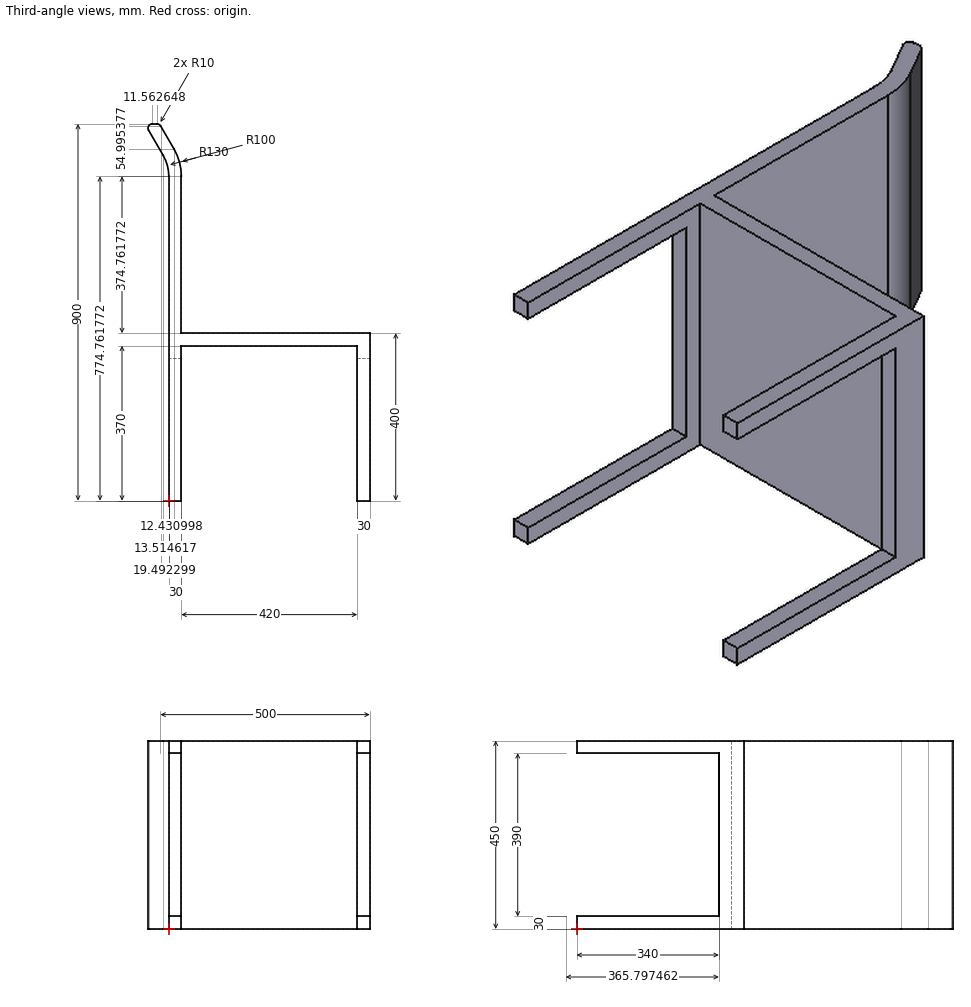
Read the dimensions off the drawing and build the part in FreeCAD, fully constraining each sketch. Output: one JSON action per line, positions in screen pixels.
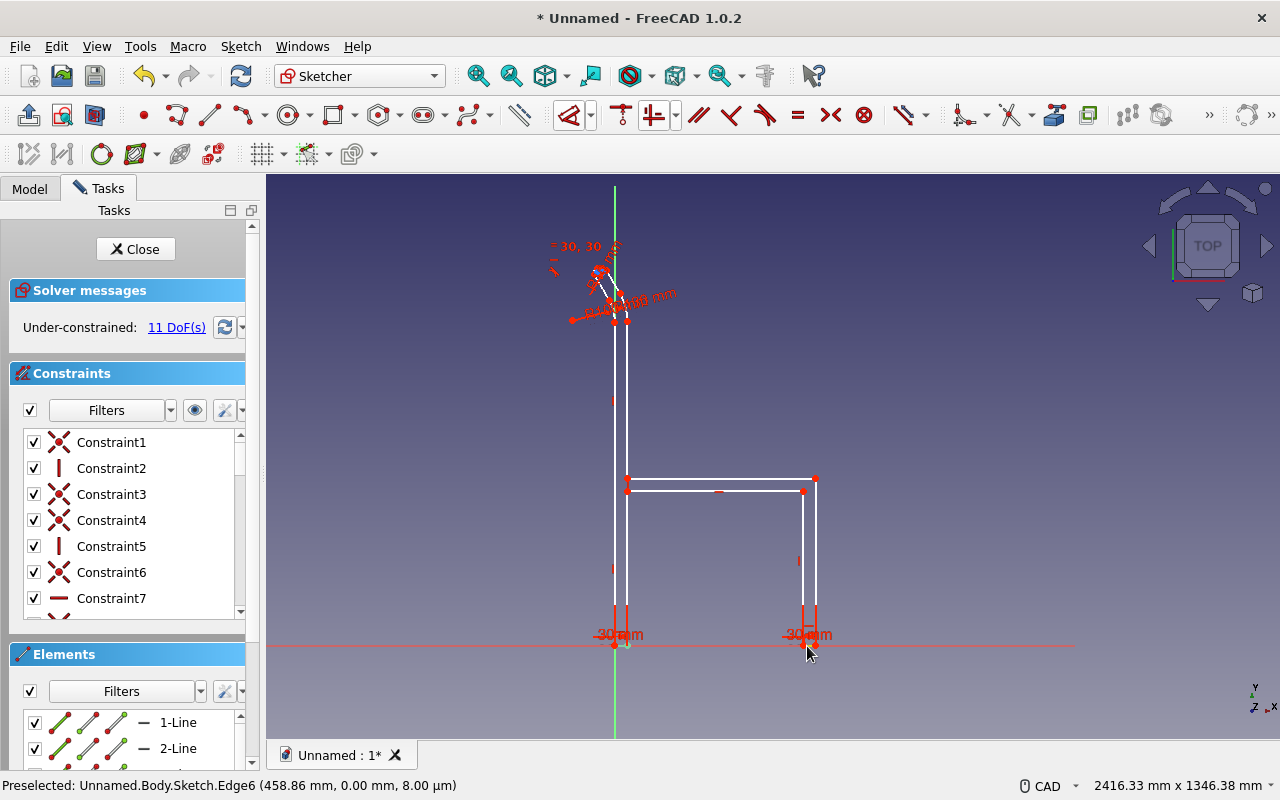
{"action": "left_click", "coordinate": [627, 599]}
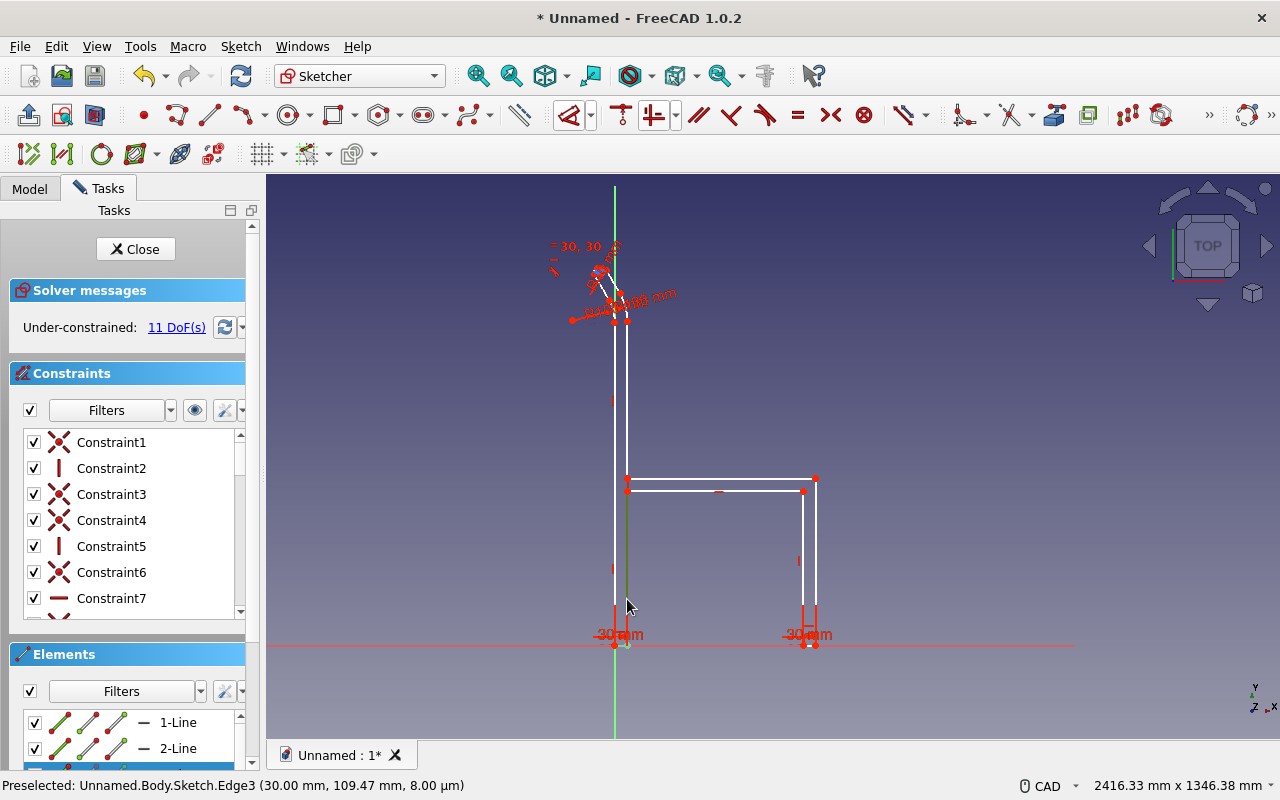
{"action": "left_click", "coordinate": [590, 116]}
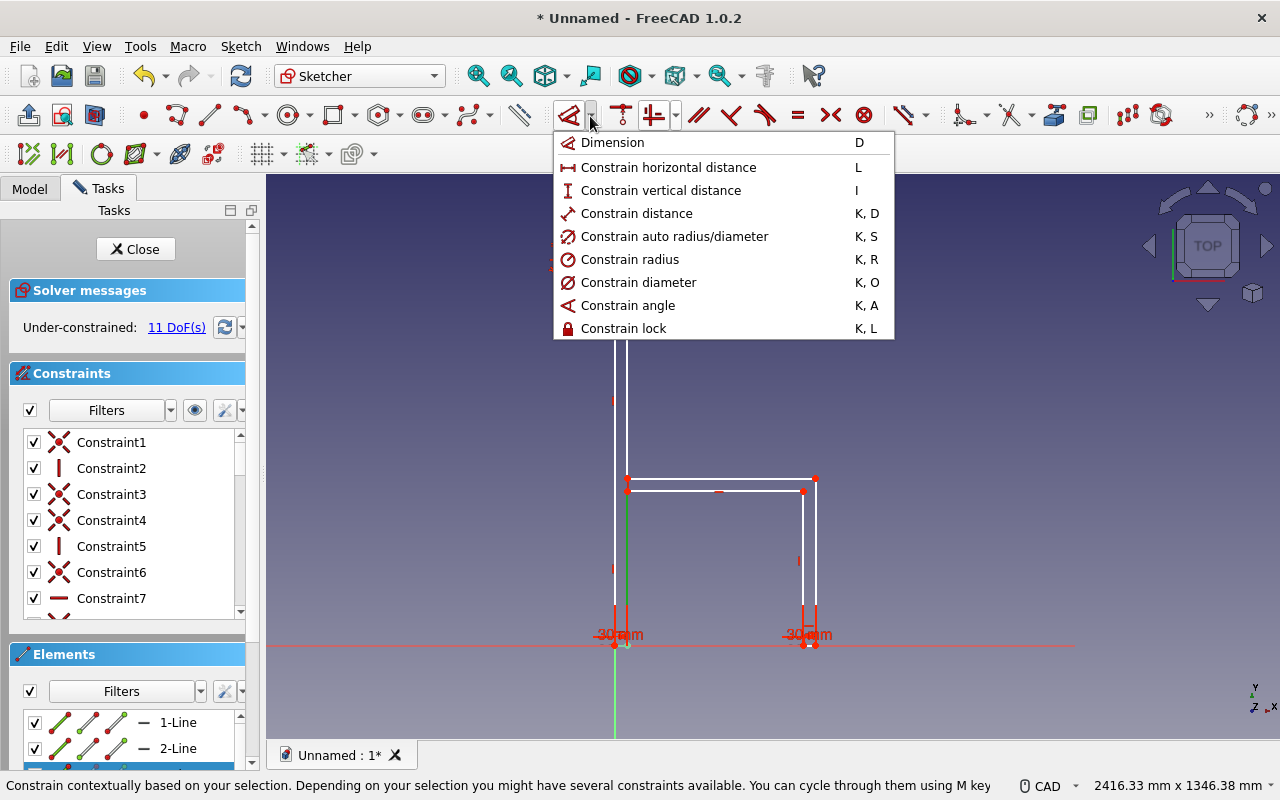
{"action": "left_click", "coordinate": [724, 190]}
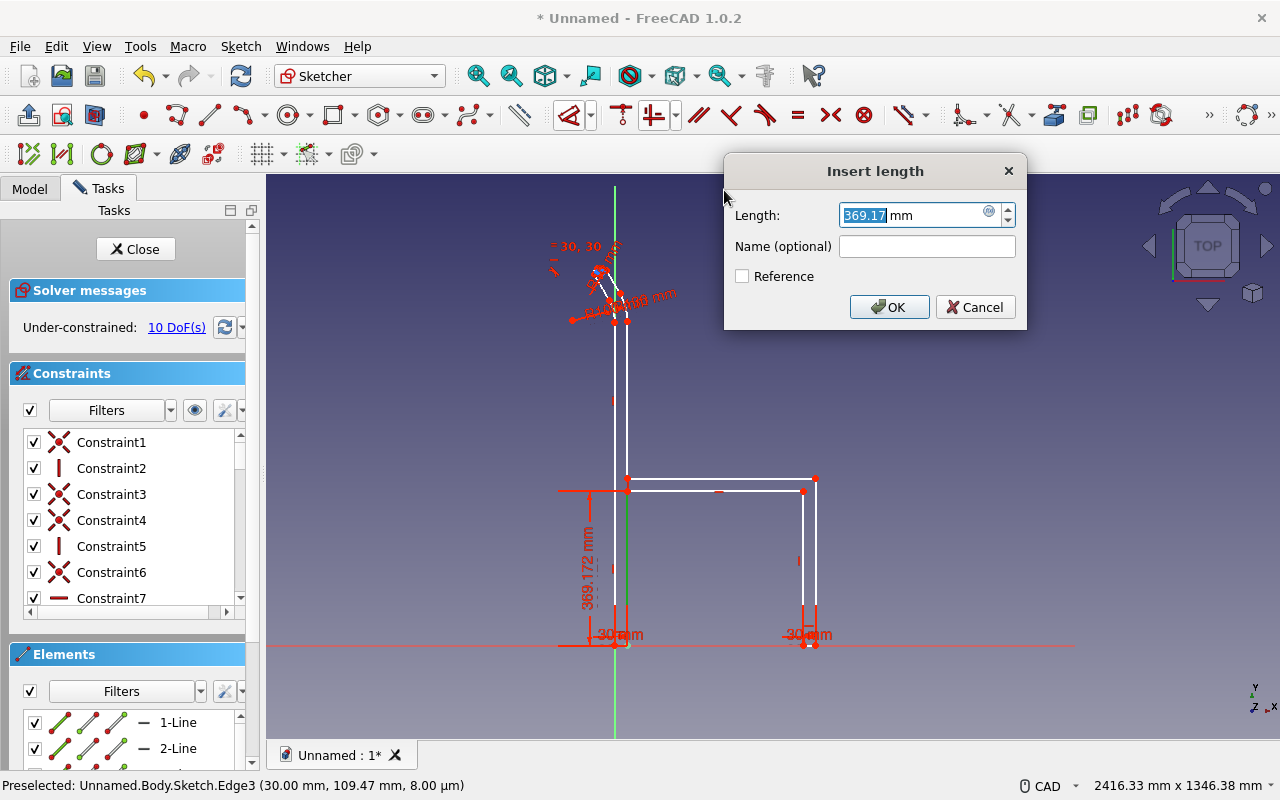
{"action": "type", "text": "370"}
{"action": "key", "text": "Return"}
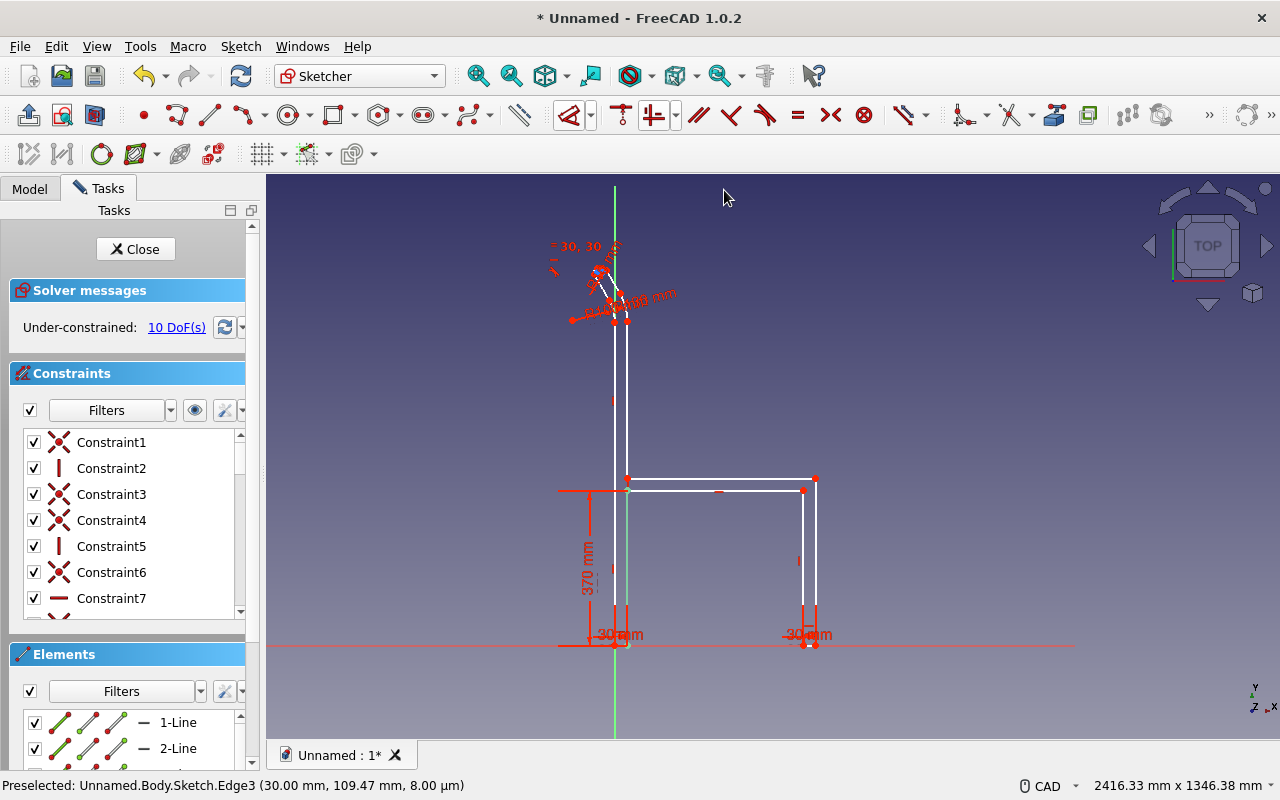
{"action": "left_click", "coordinate": [680, 491]}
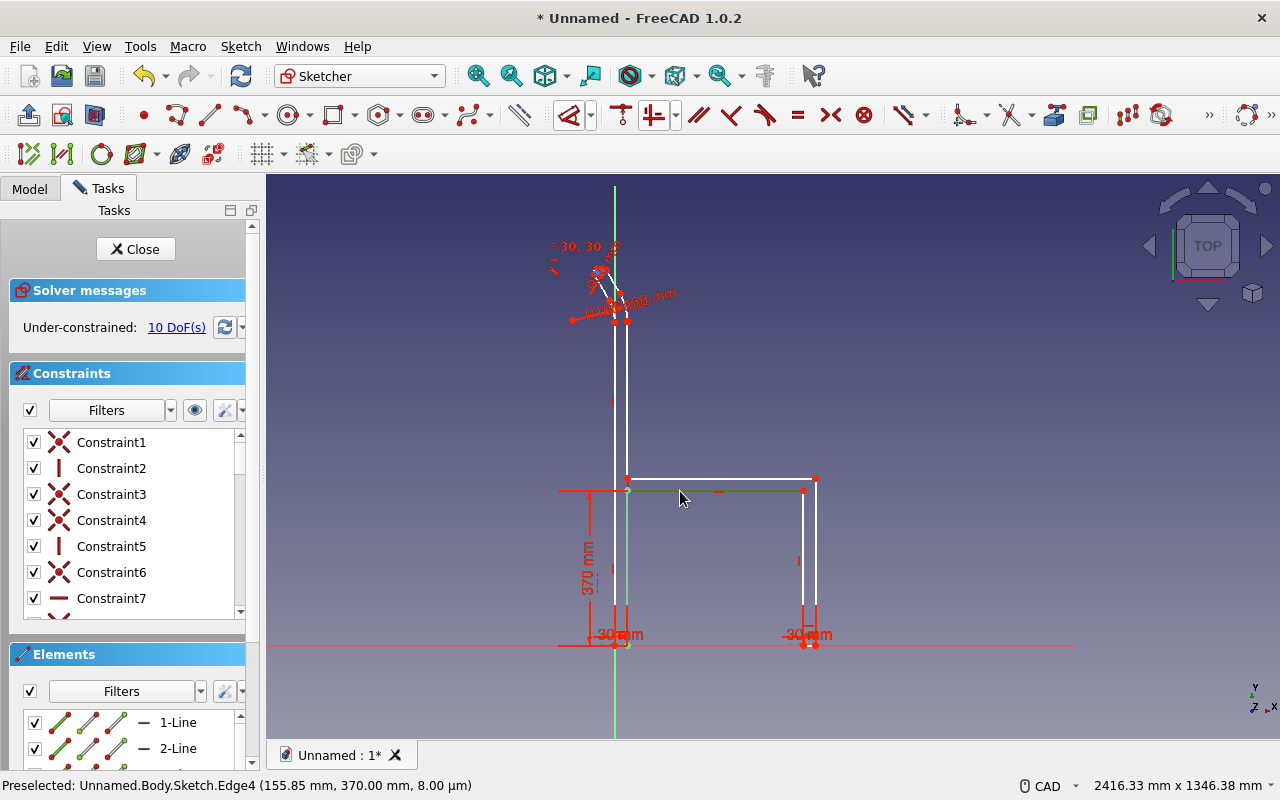
{"action": "left_click", "coordinate": [590, 116]}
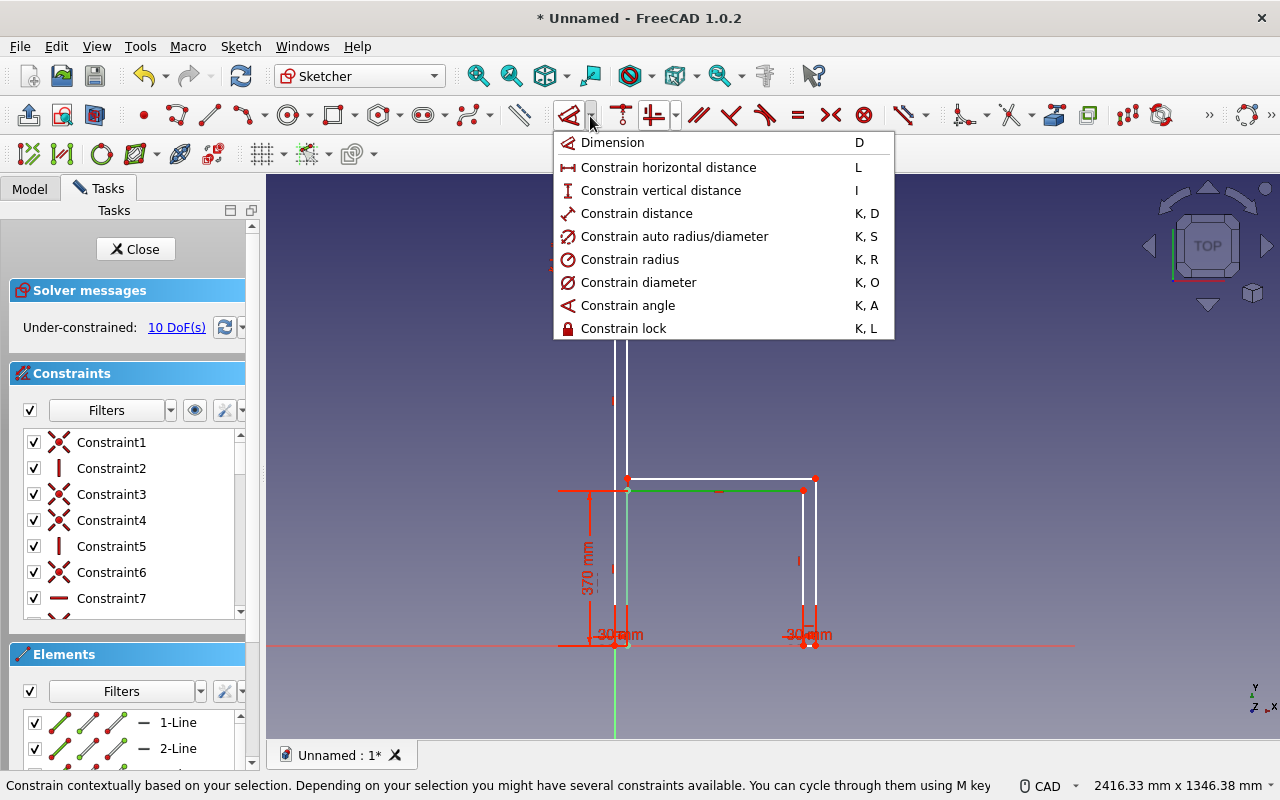
{"action": "left_click", "coordinate": [724, 168]}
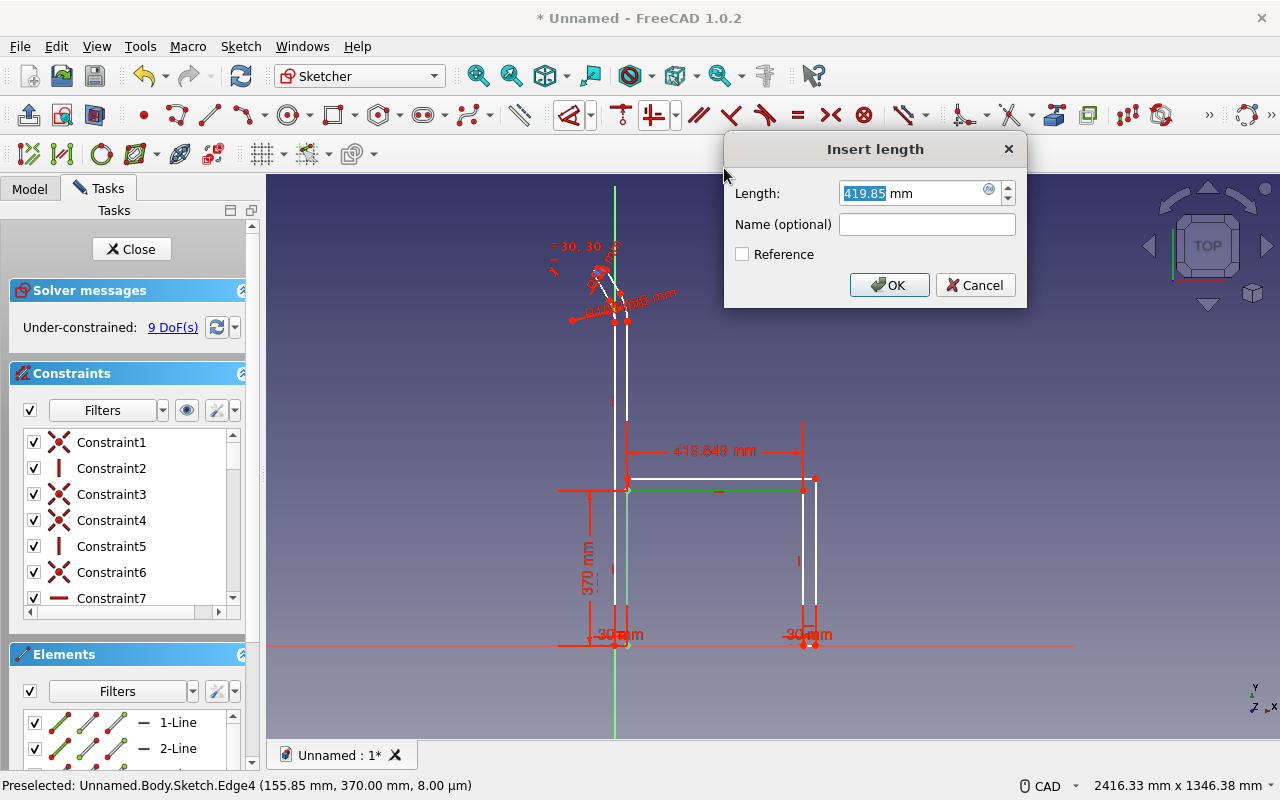
{"action": "type", "text": "420"}
{"action": "key", "text": "Return"}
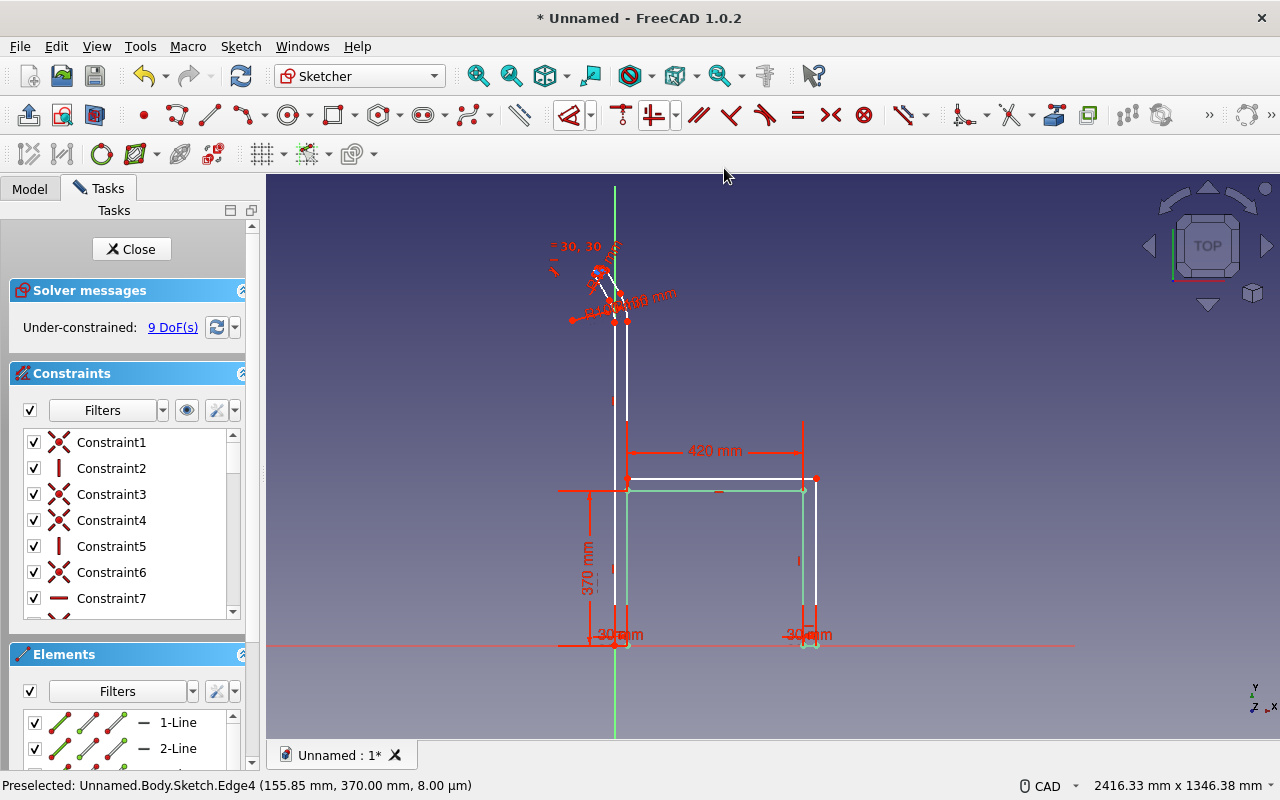
{"action": "left_click", "coordinate": [816, 596]}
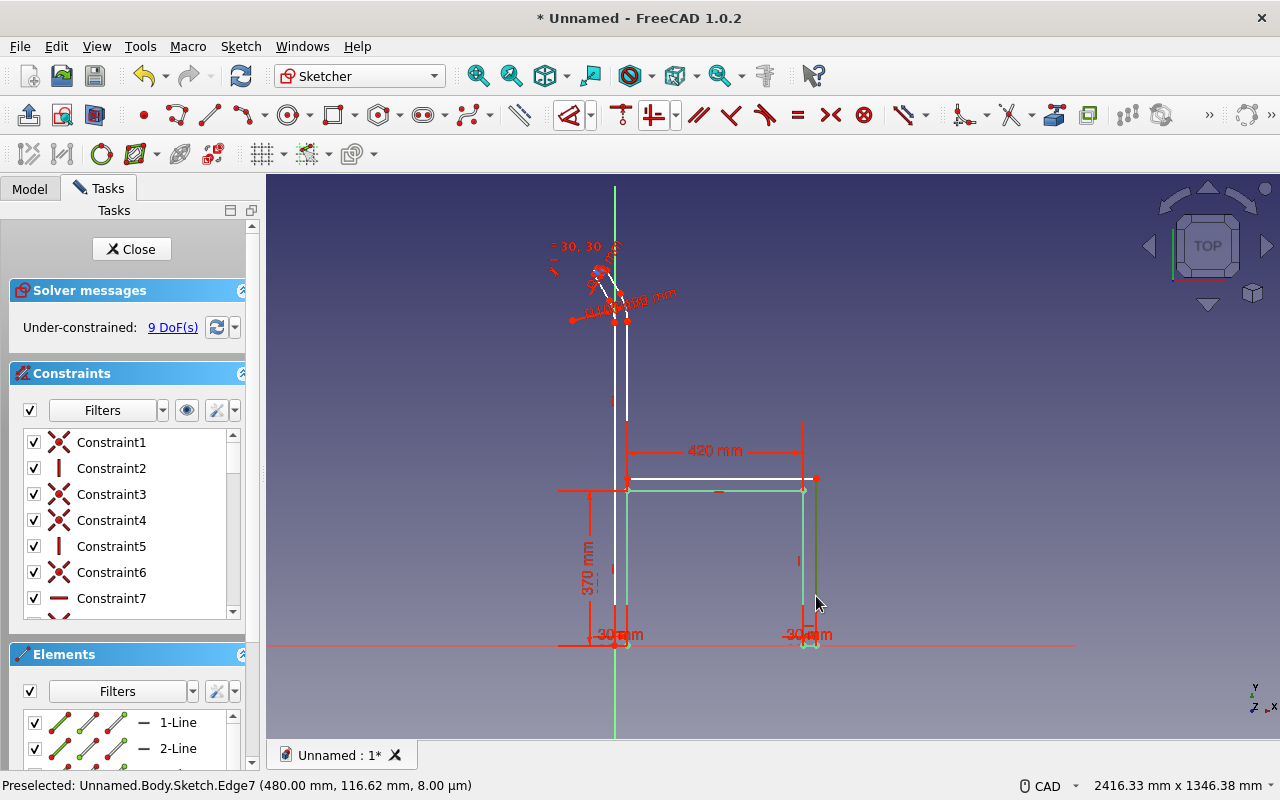
{"action": "left_click", "coordinate": [590, 116]}